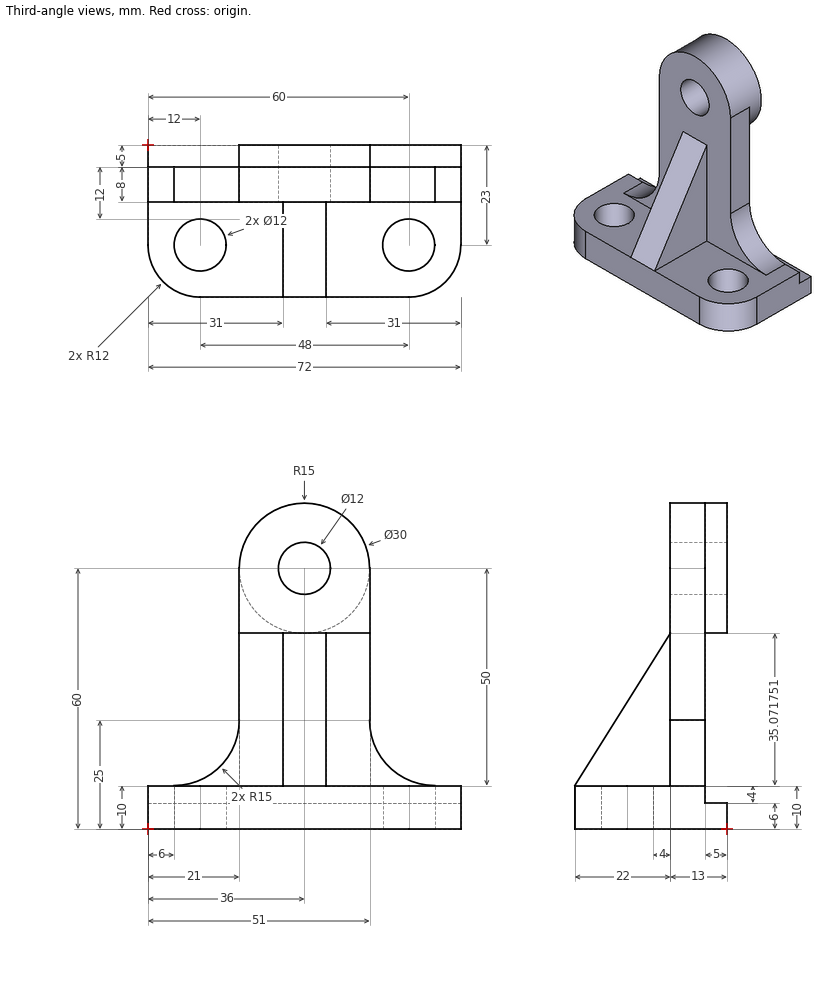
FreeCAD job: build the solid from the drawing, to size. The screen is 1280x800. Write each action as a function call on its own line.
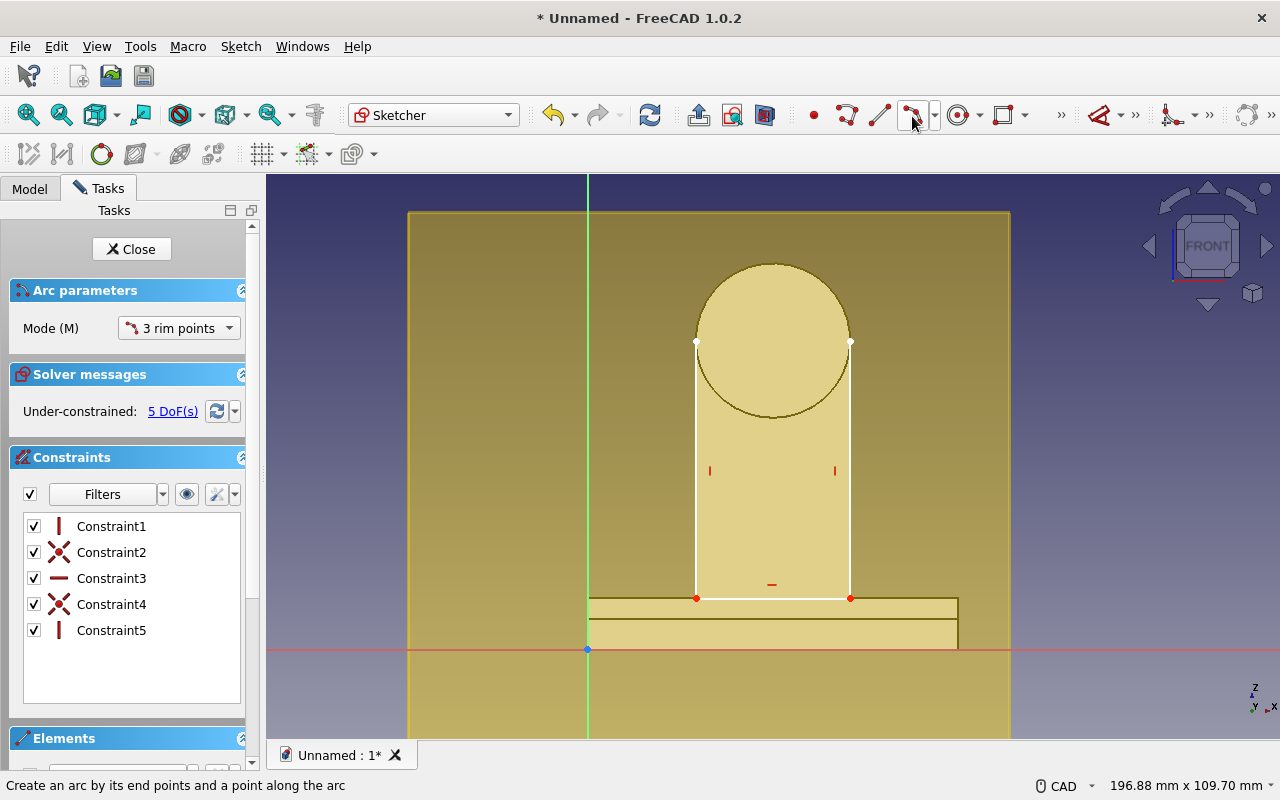
click(850, 342)
click(696, 342)
click(773, 263)
key(Escape)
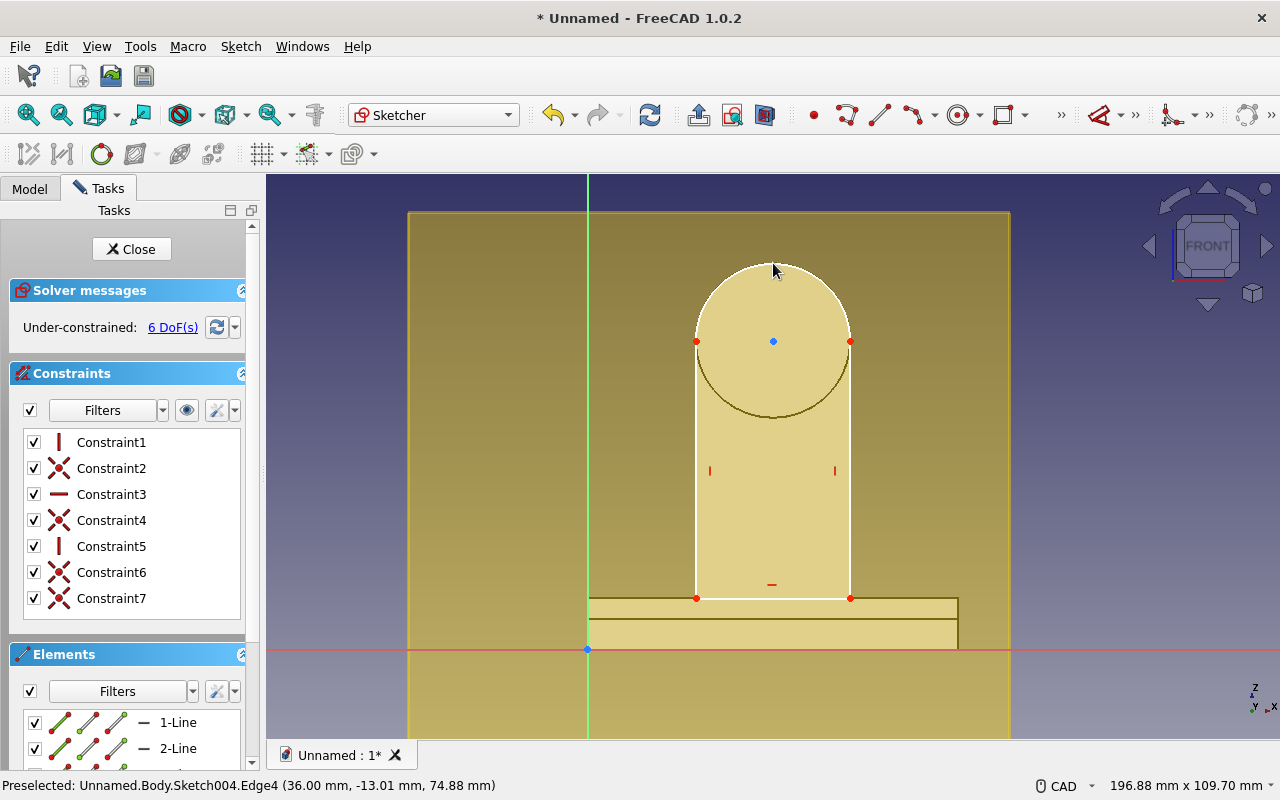
click(696, 419)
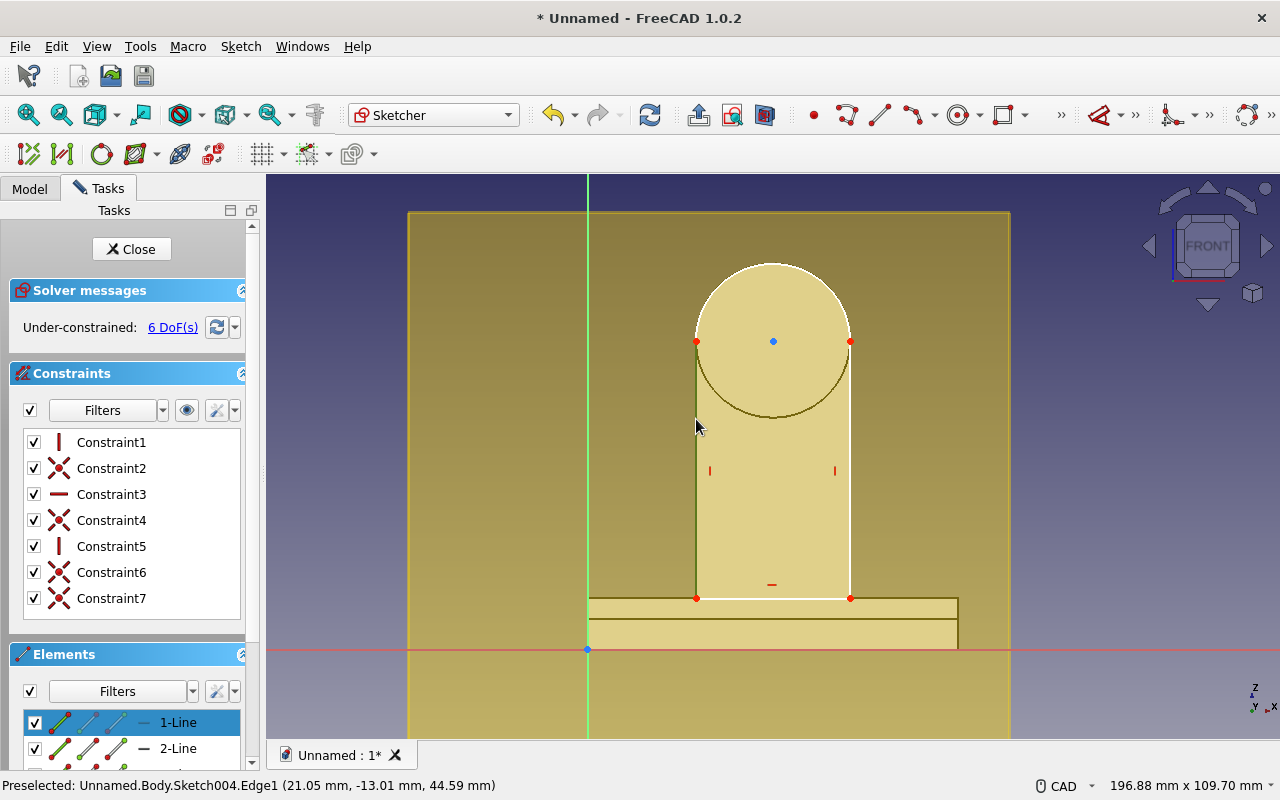
click(819, 279)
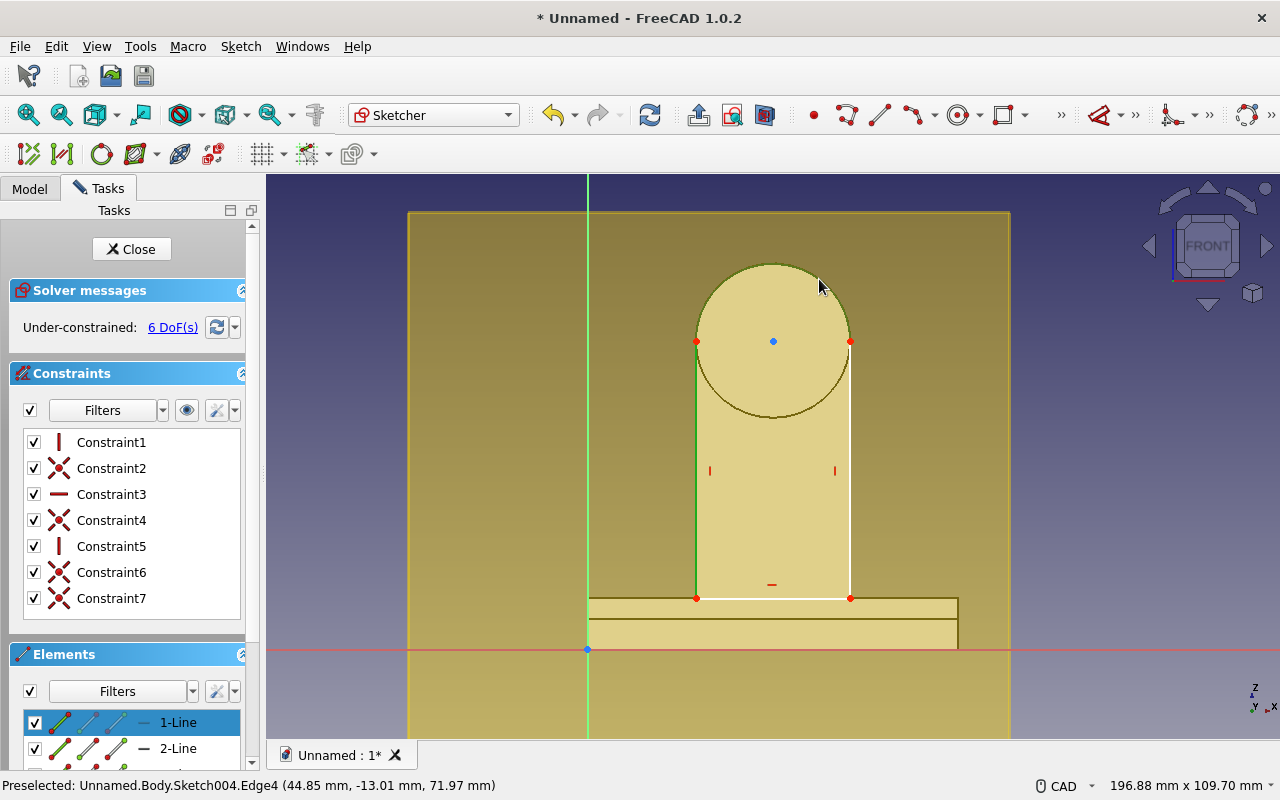
key(t)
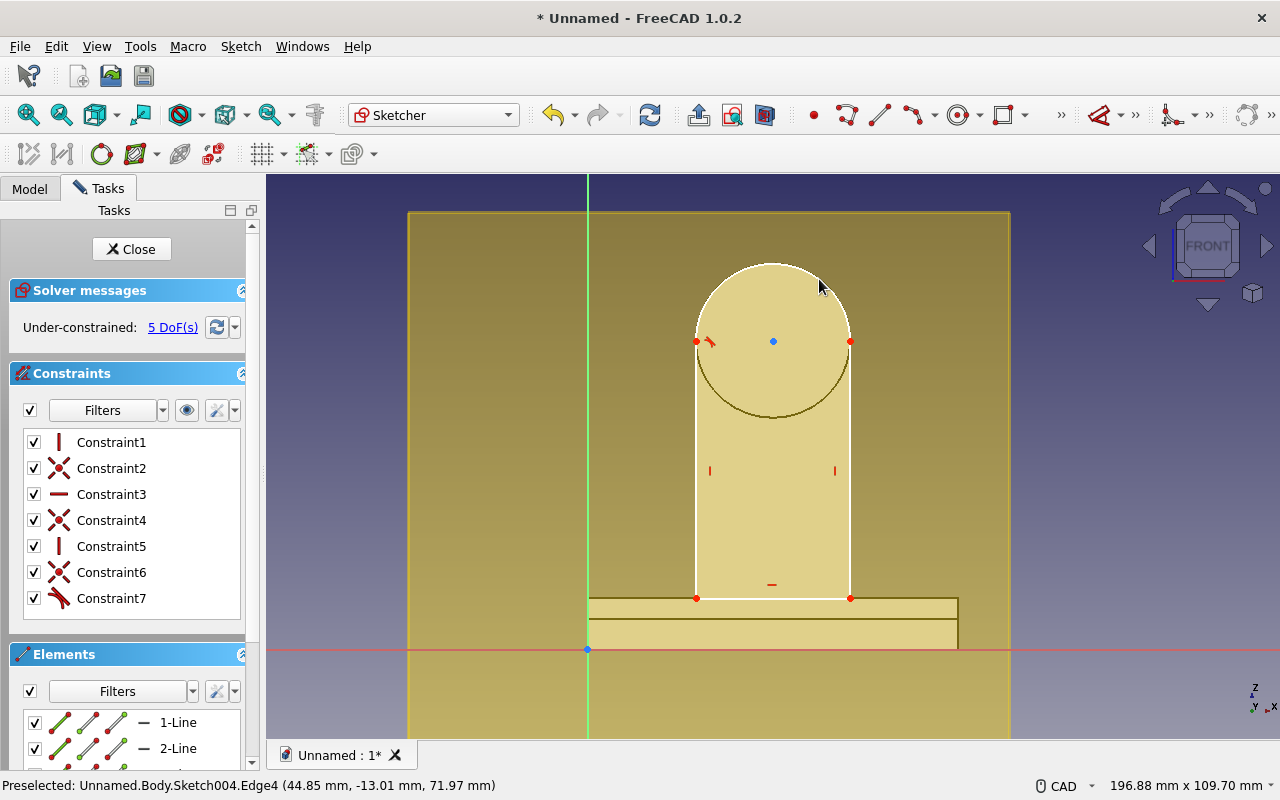
click(850, 522)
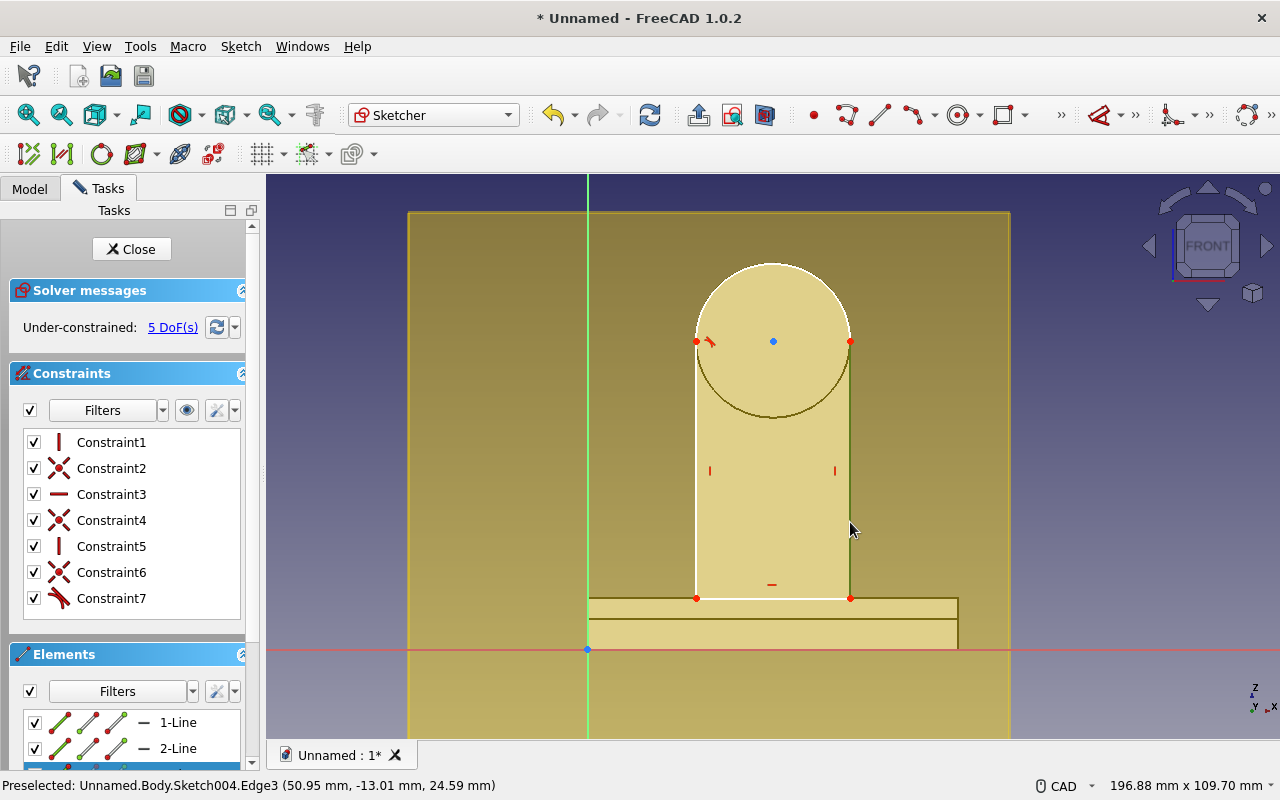
click(819, 279)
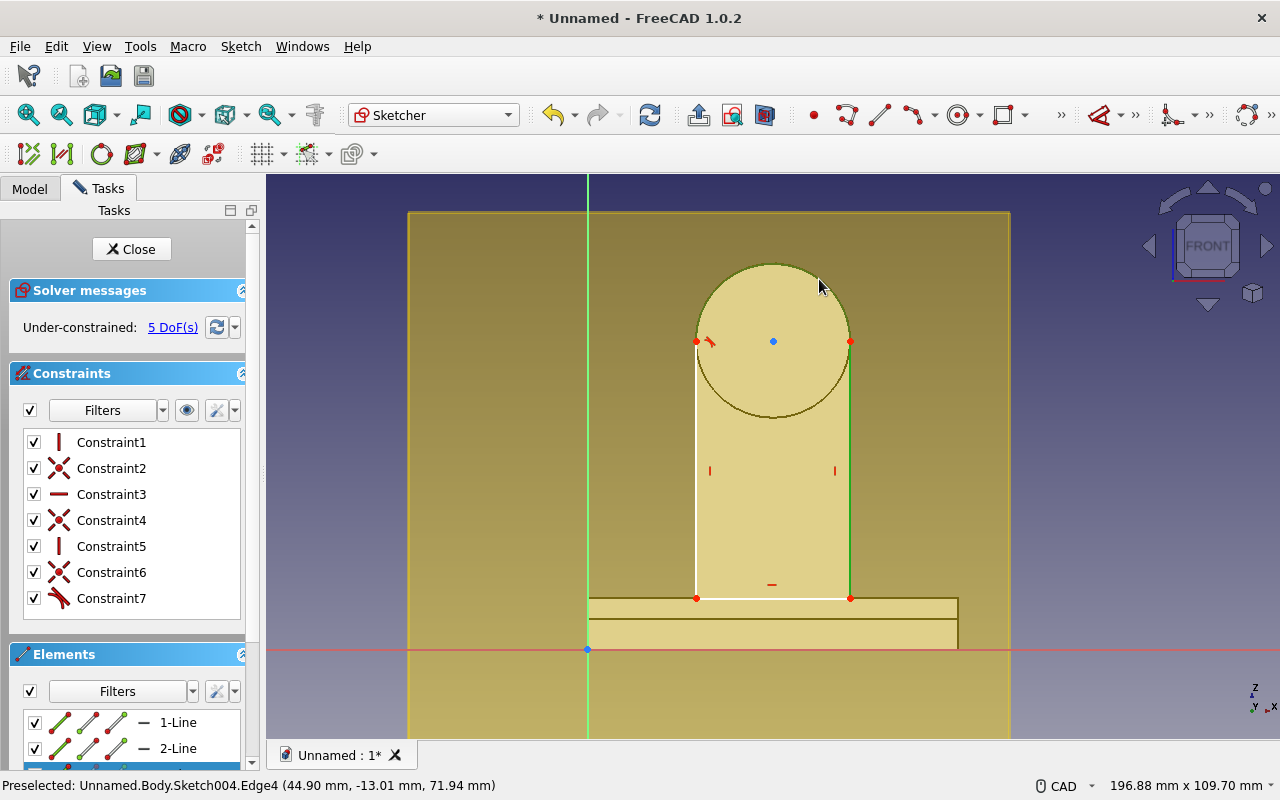
key(t)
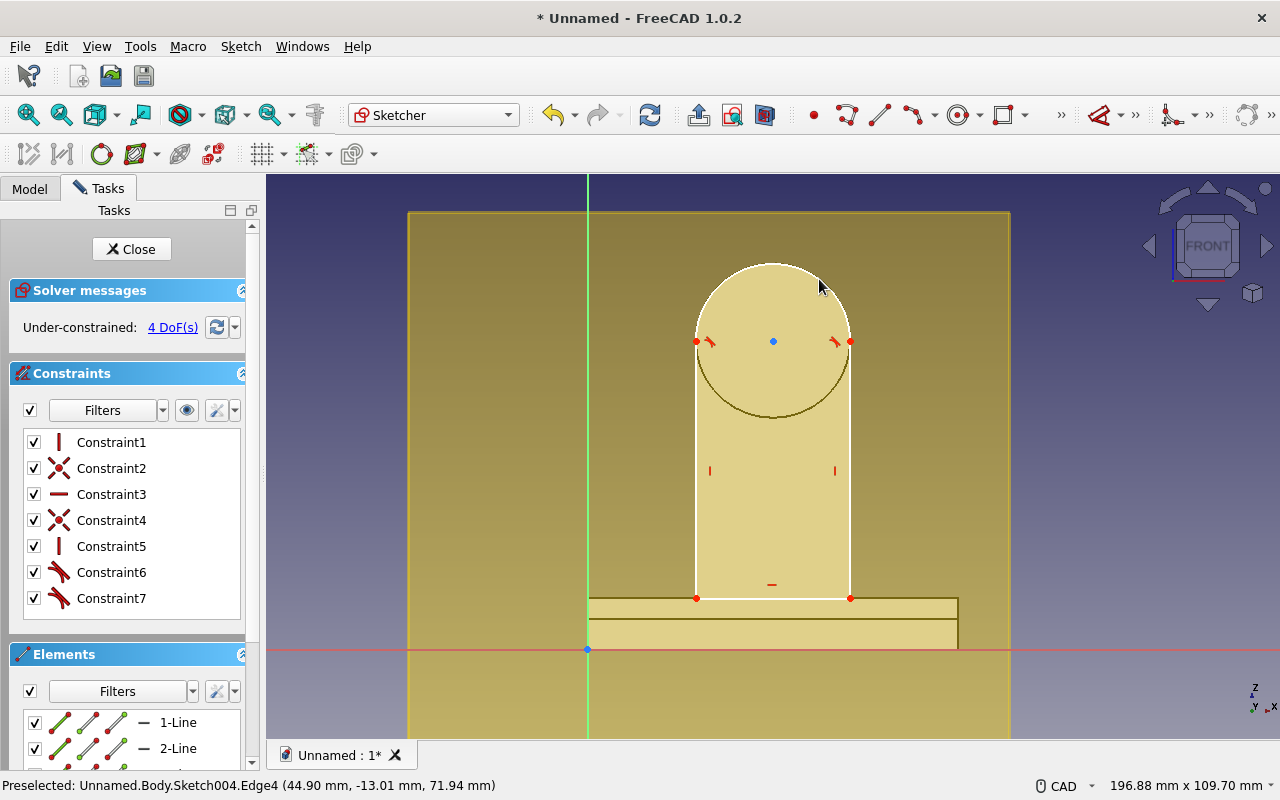
key(d)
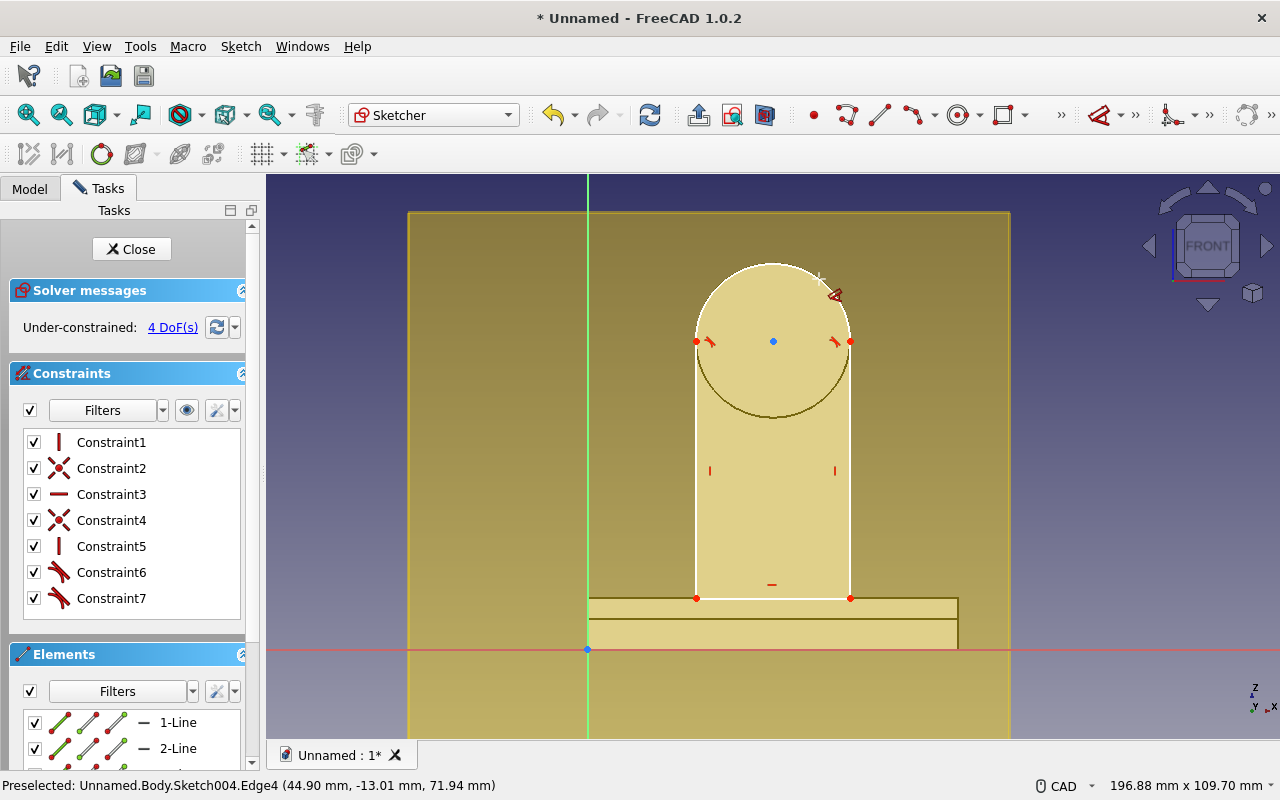
click(818, 279)
click(837, 253)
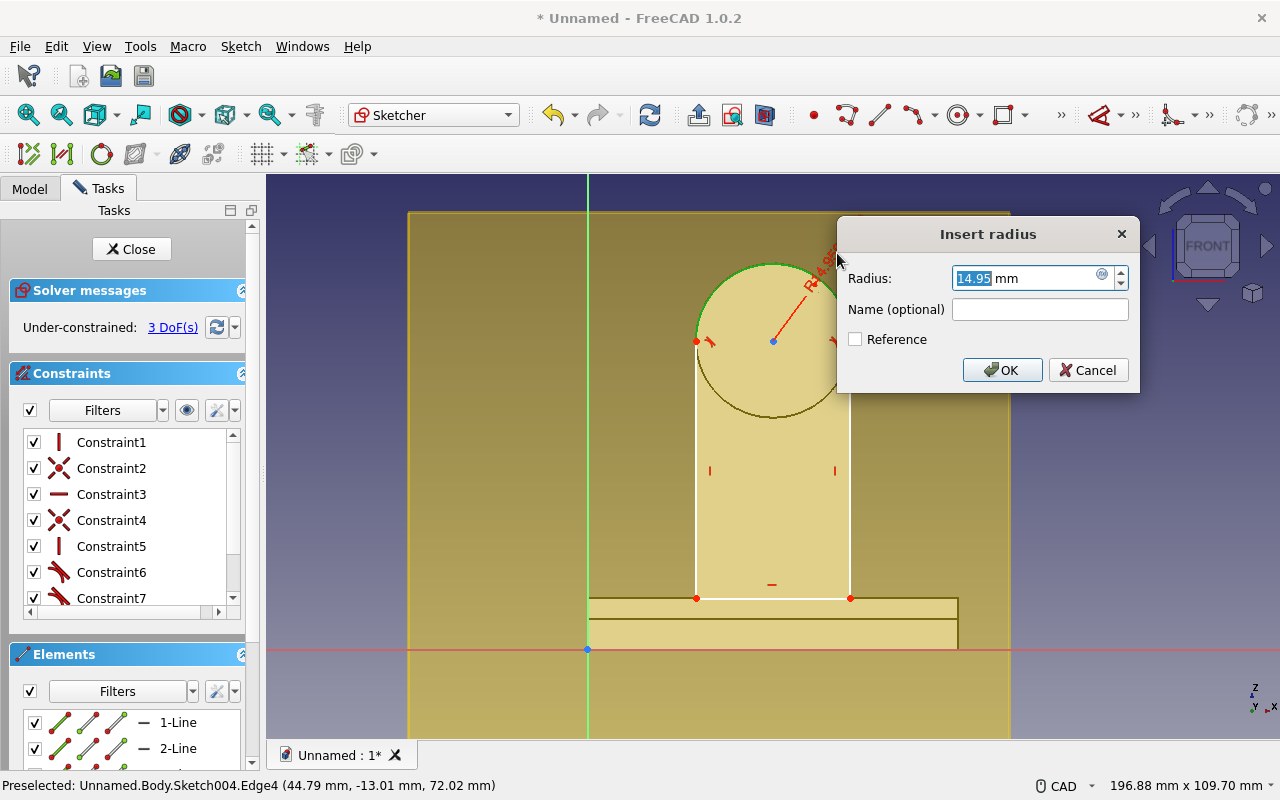
text(15)
key(Return)